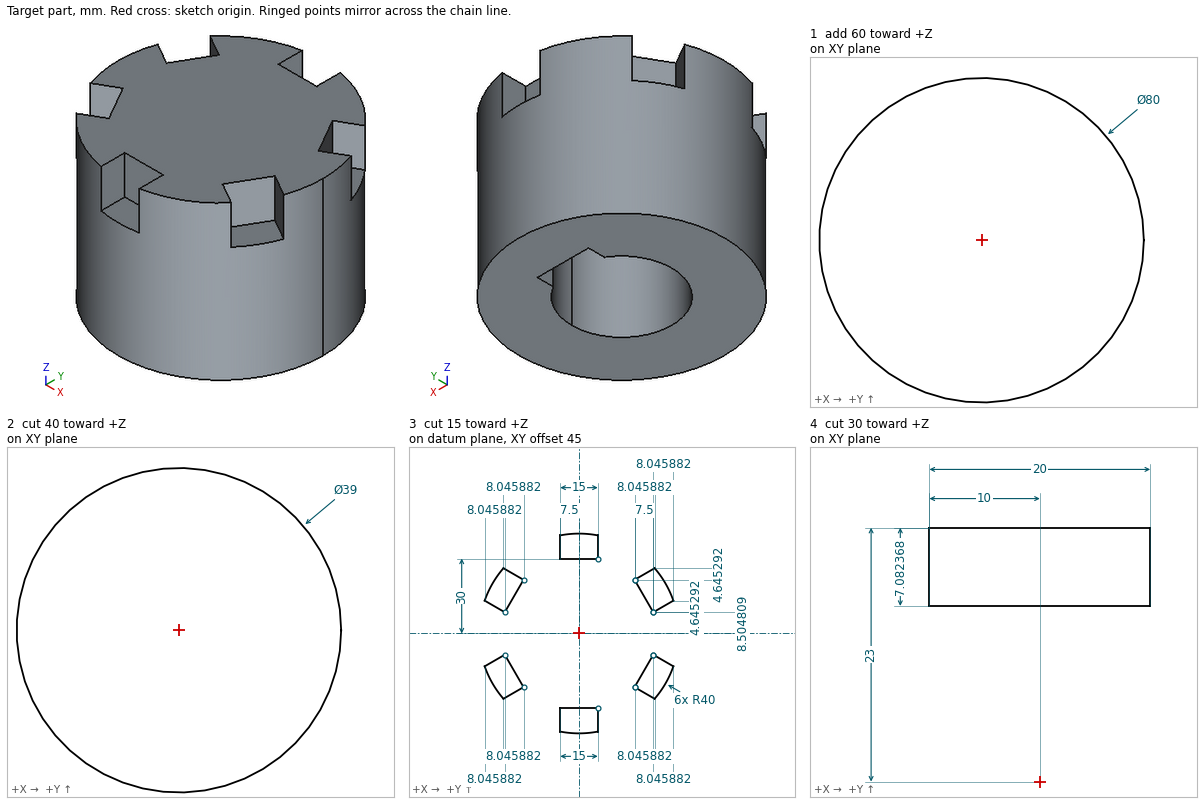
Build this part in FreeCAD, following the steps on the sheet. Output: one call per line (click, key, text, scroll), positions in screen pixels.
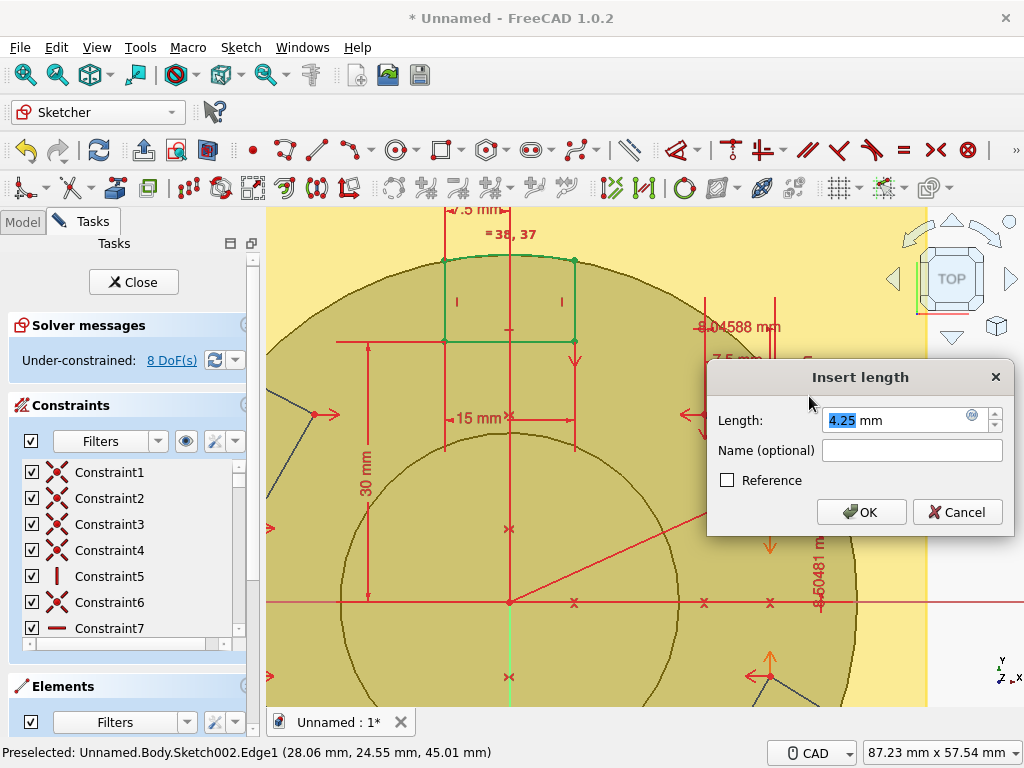
text(4.645292)
key(Return)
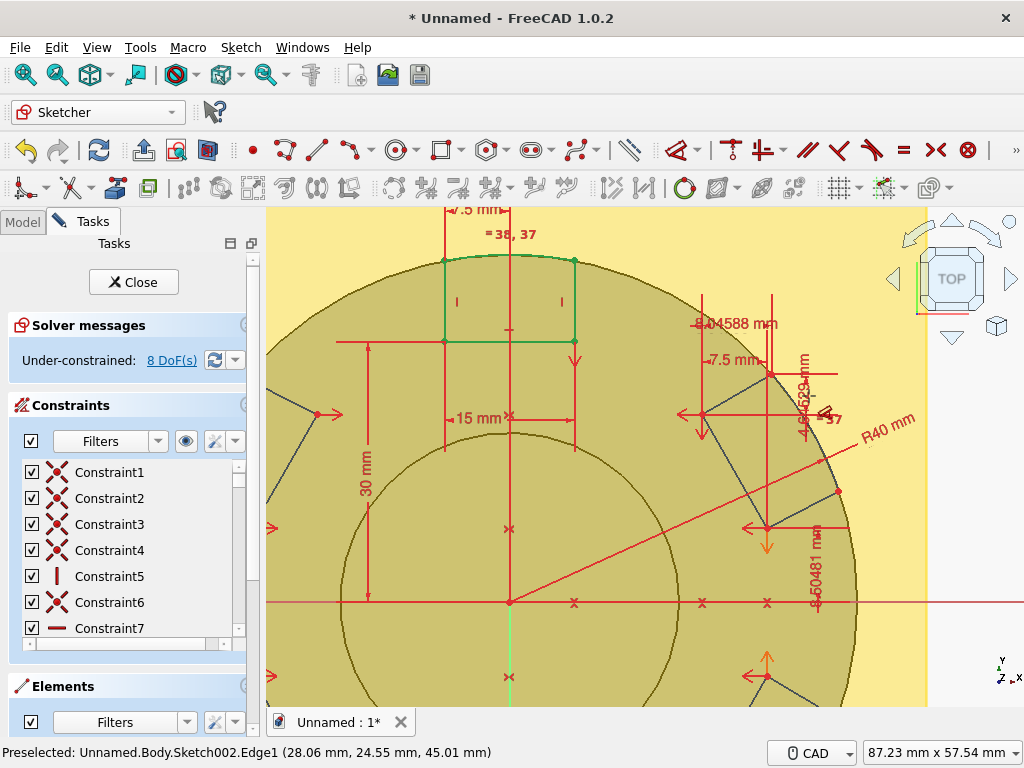
click(789, 517)
click(803, 457)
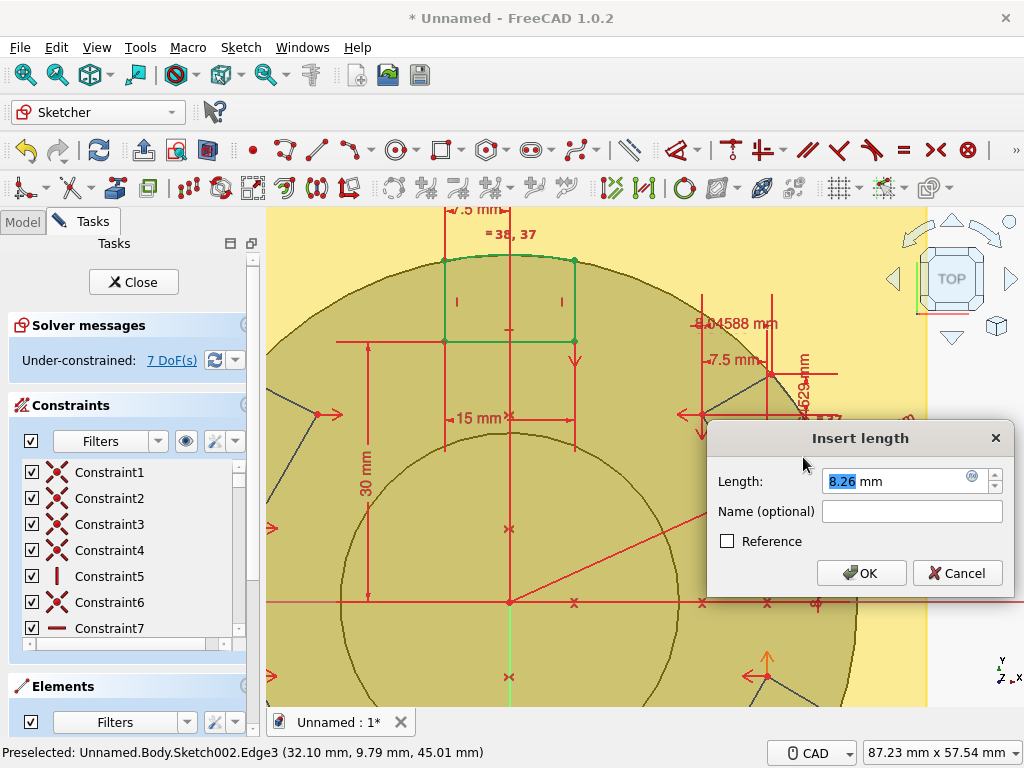
text(8.045882)
key(Return)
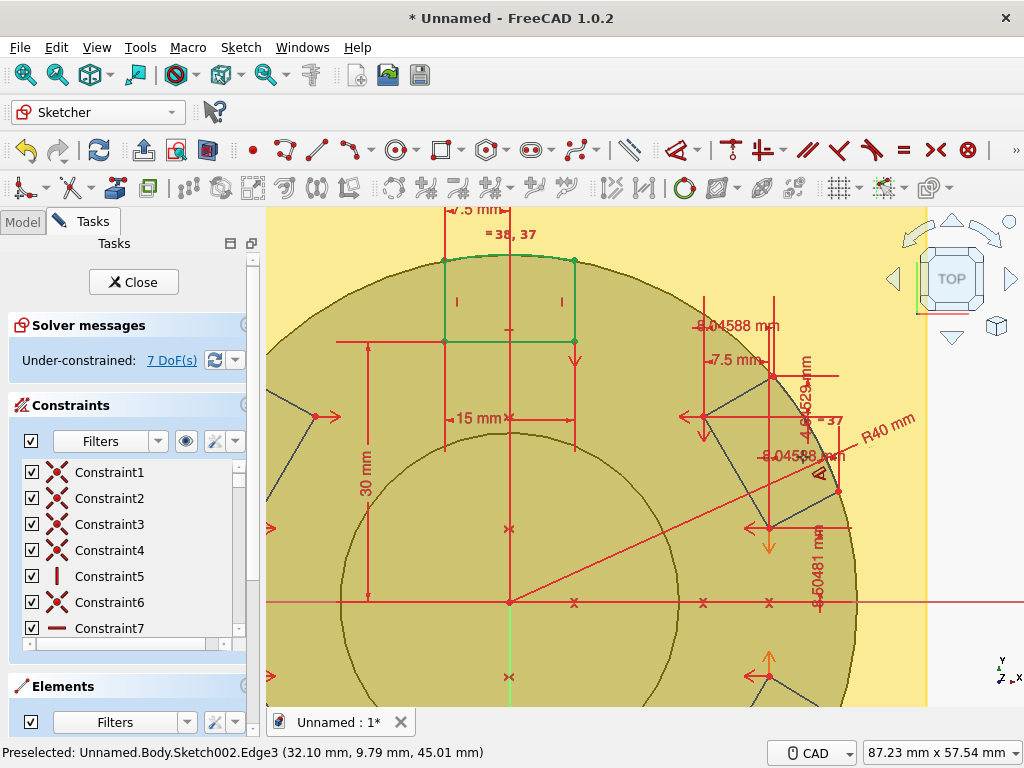
click(790, 517)
click(735, 510)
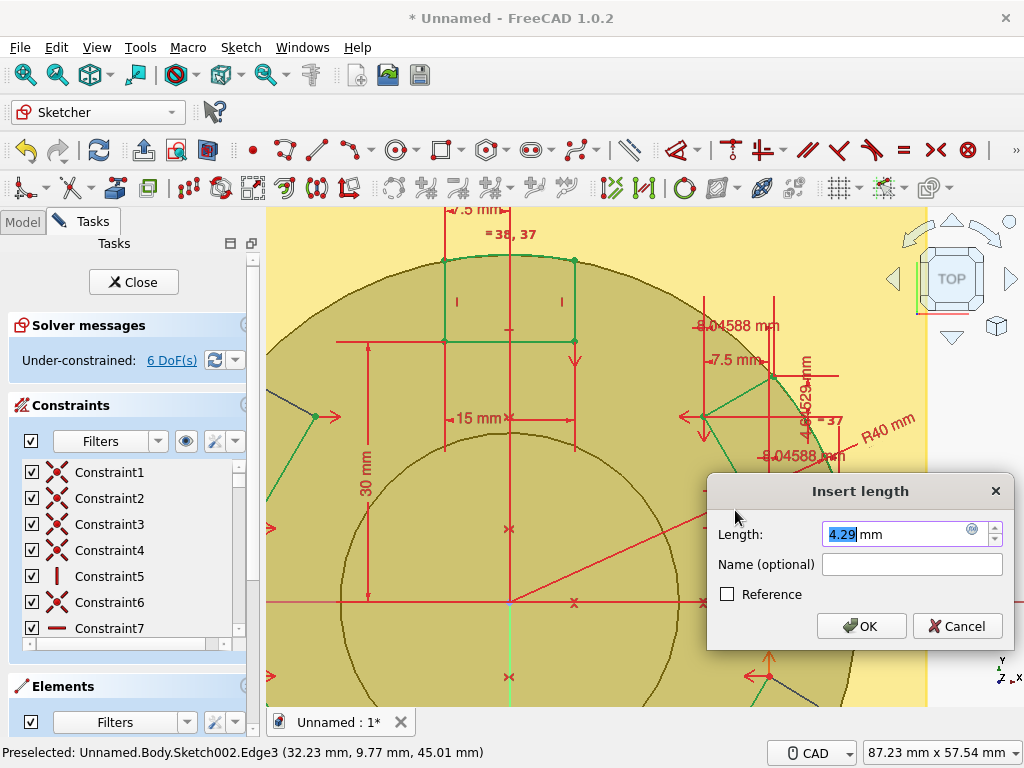
text(4.645292)
key(Return)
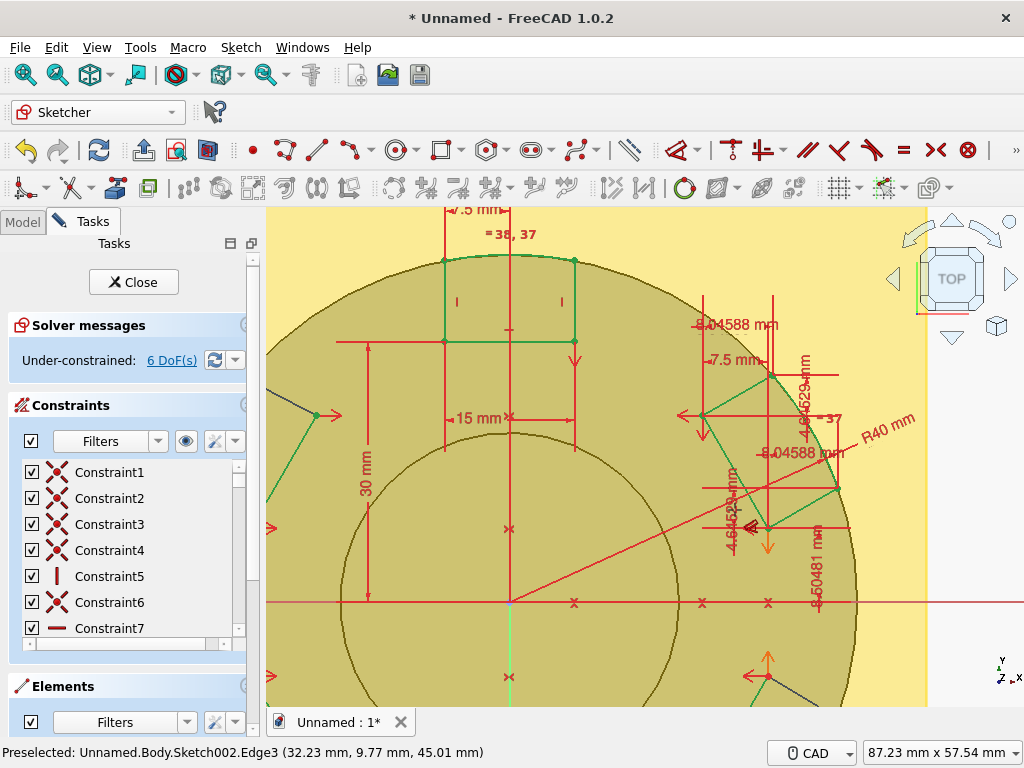
scroll(631, 338, down, 4)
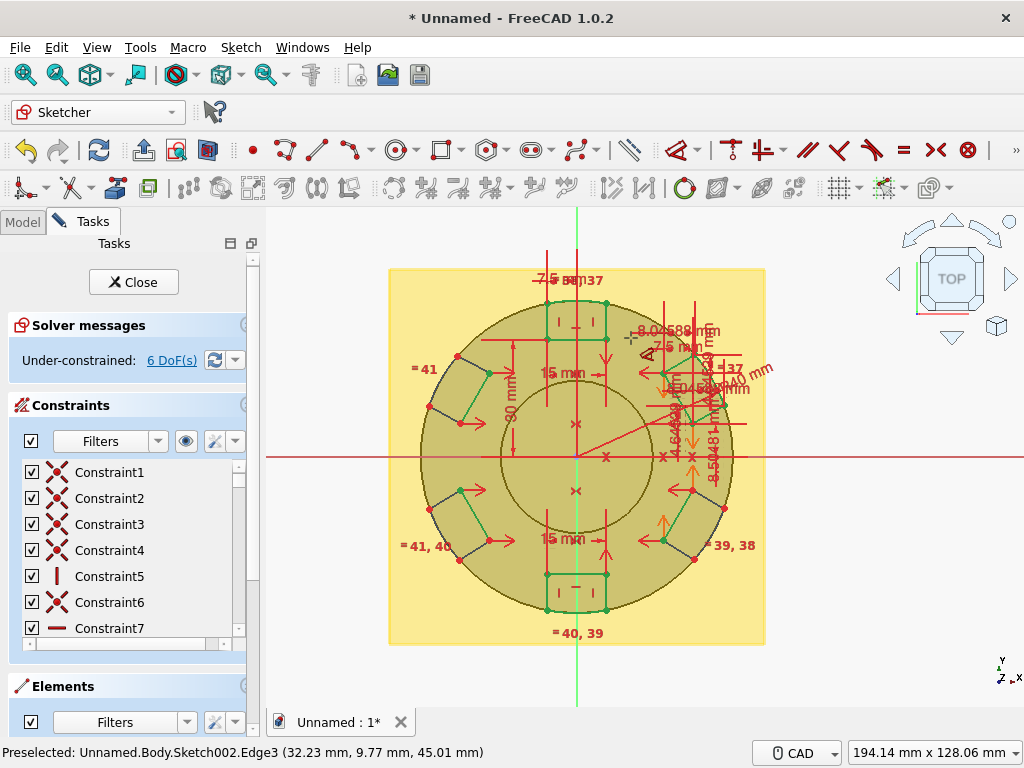
scroll(715, 503, up, 2)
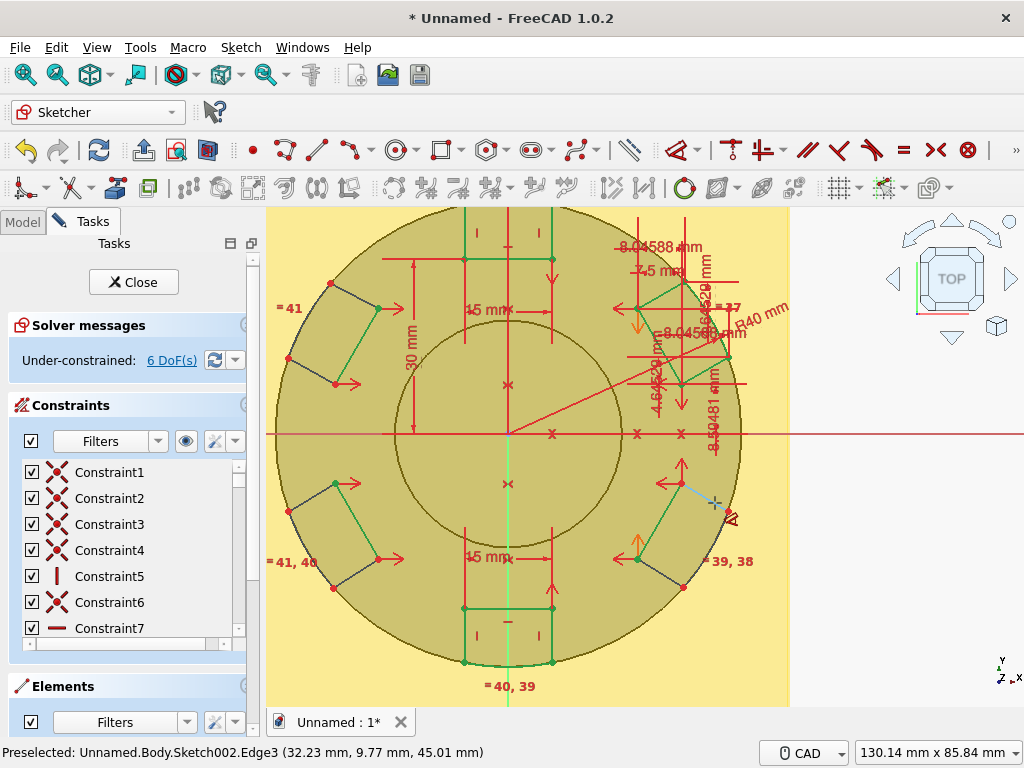
click(714, 503)
click(694, 546)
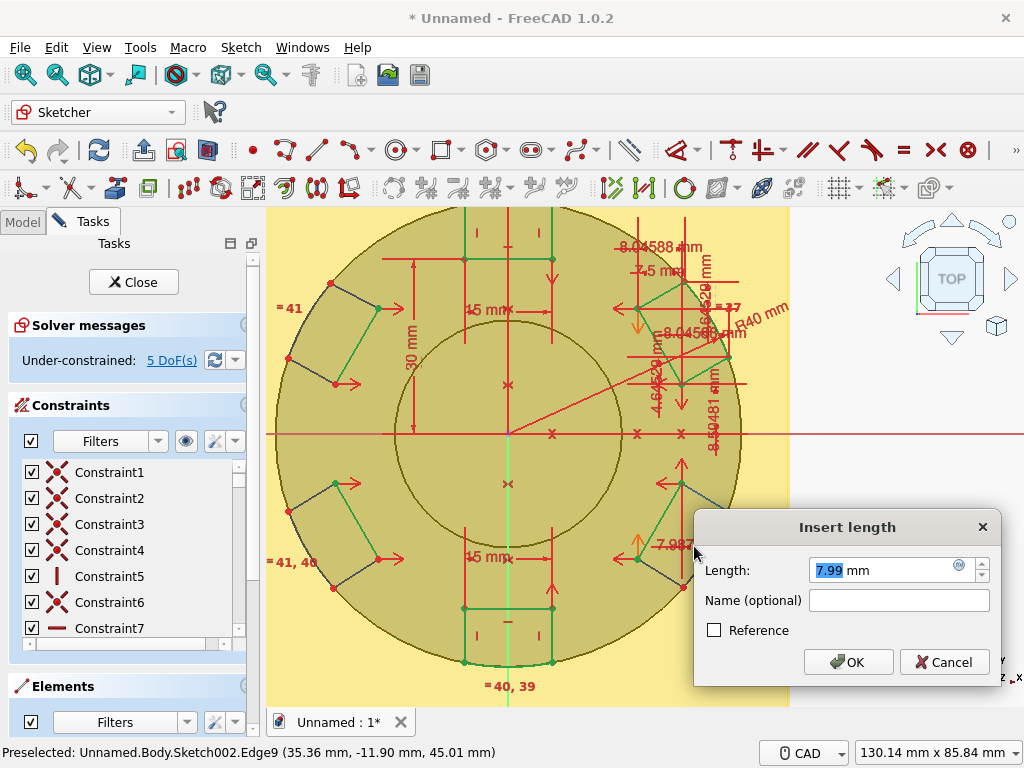
text(8.045882)
key(Return)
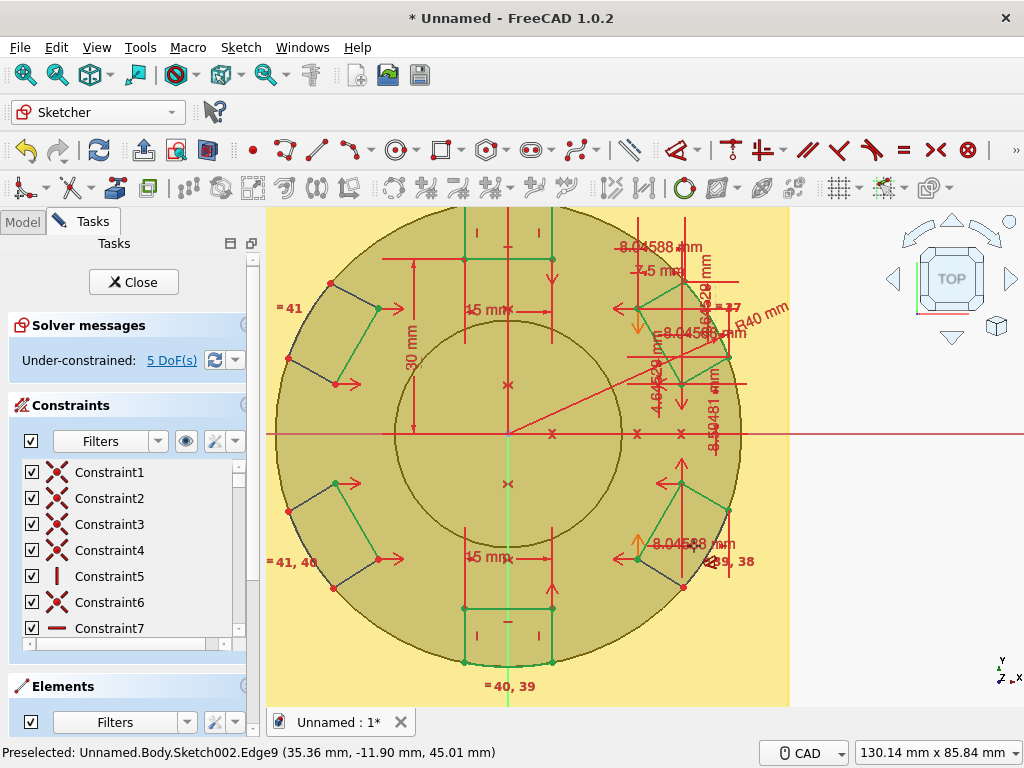
click(652, 568)
click(661, 622)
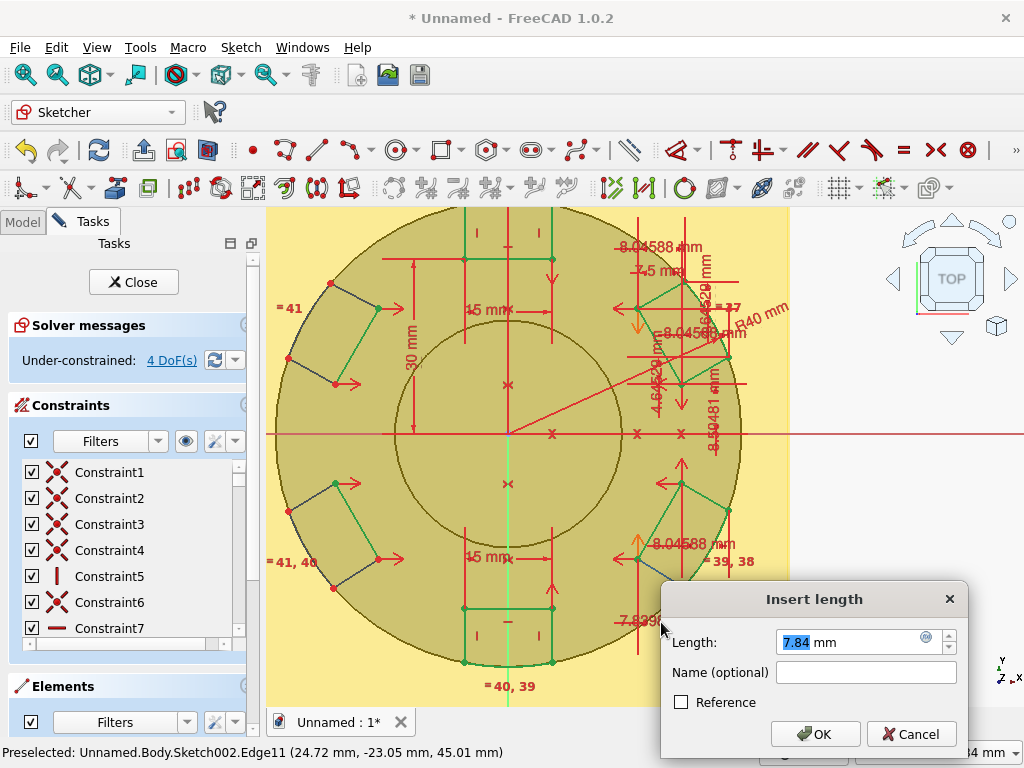
text(8.045882)
key(Return)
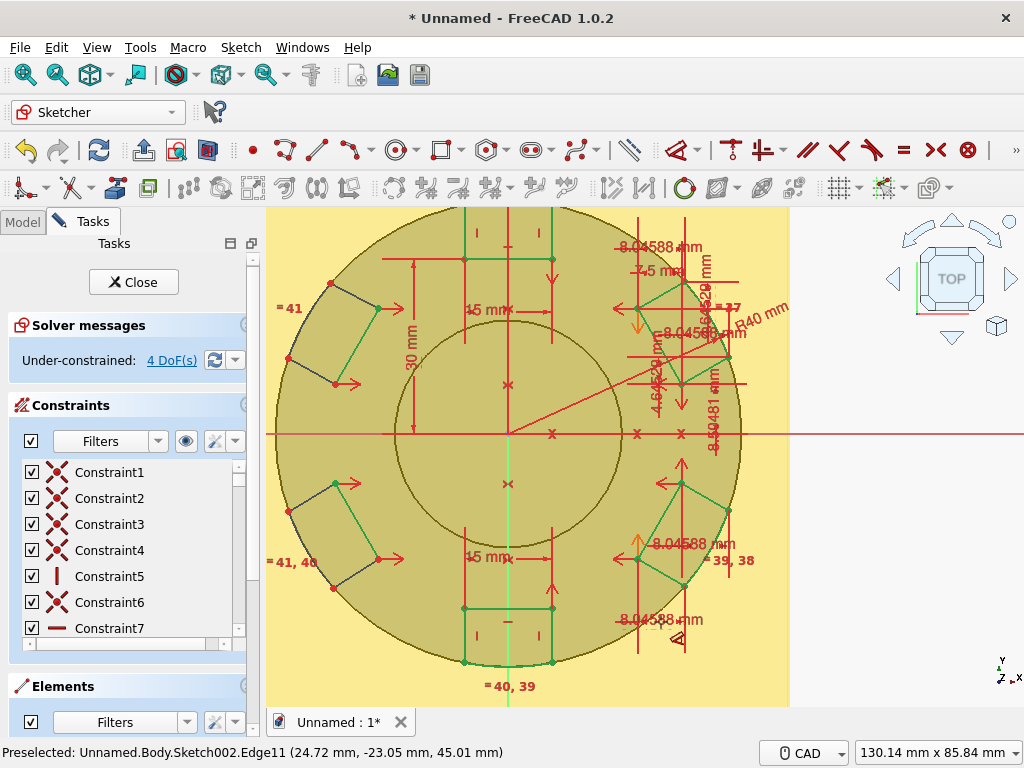
click(347, 579)
click(356, 622)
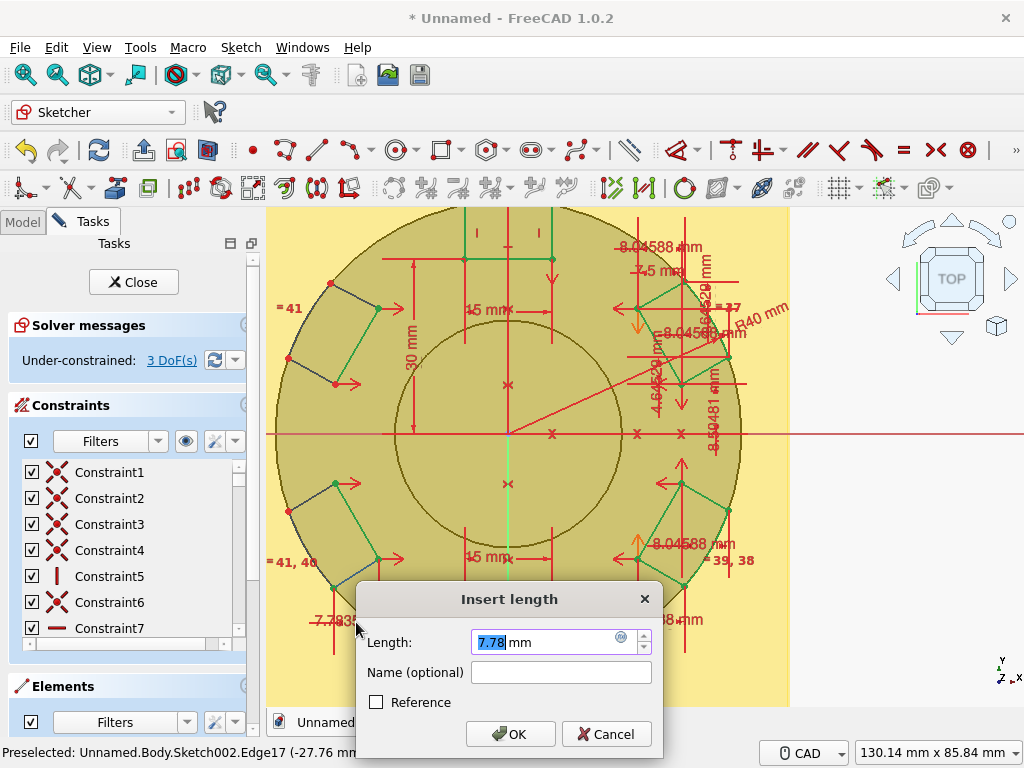
text(8.045882)
key(Return)